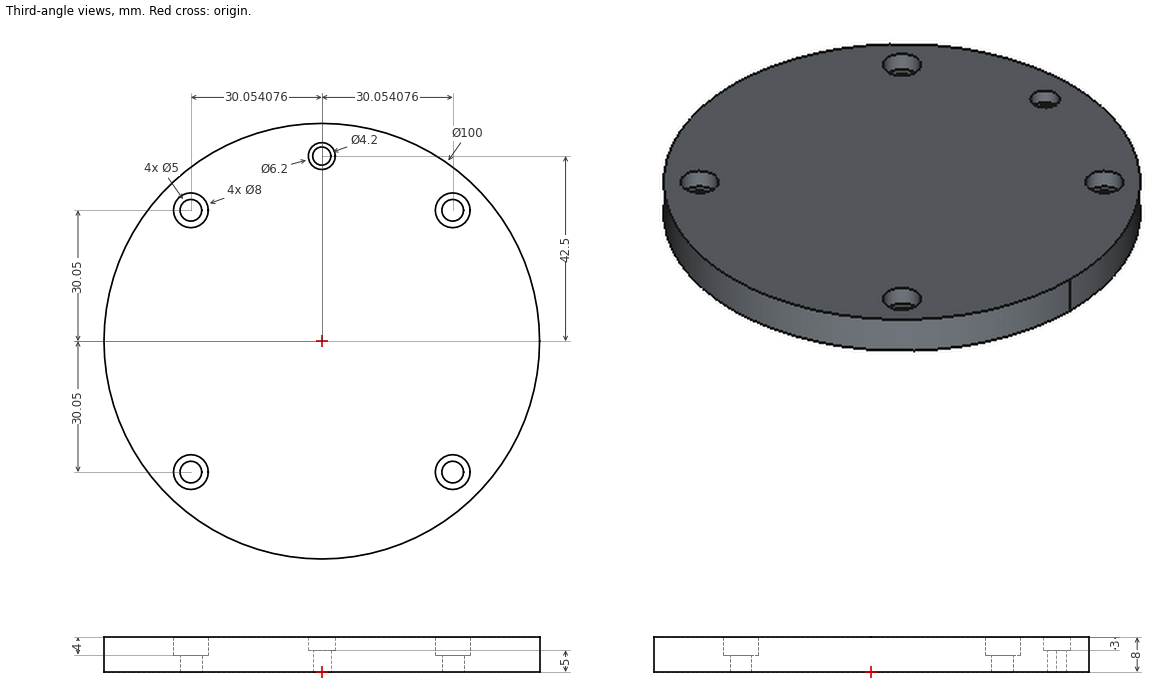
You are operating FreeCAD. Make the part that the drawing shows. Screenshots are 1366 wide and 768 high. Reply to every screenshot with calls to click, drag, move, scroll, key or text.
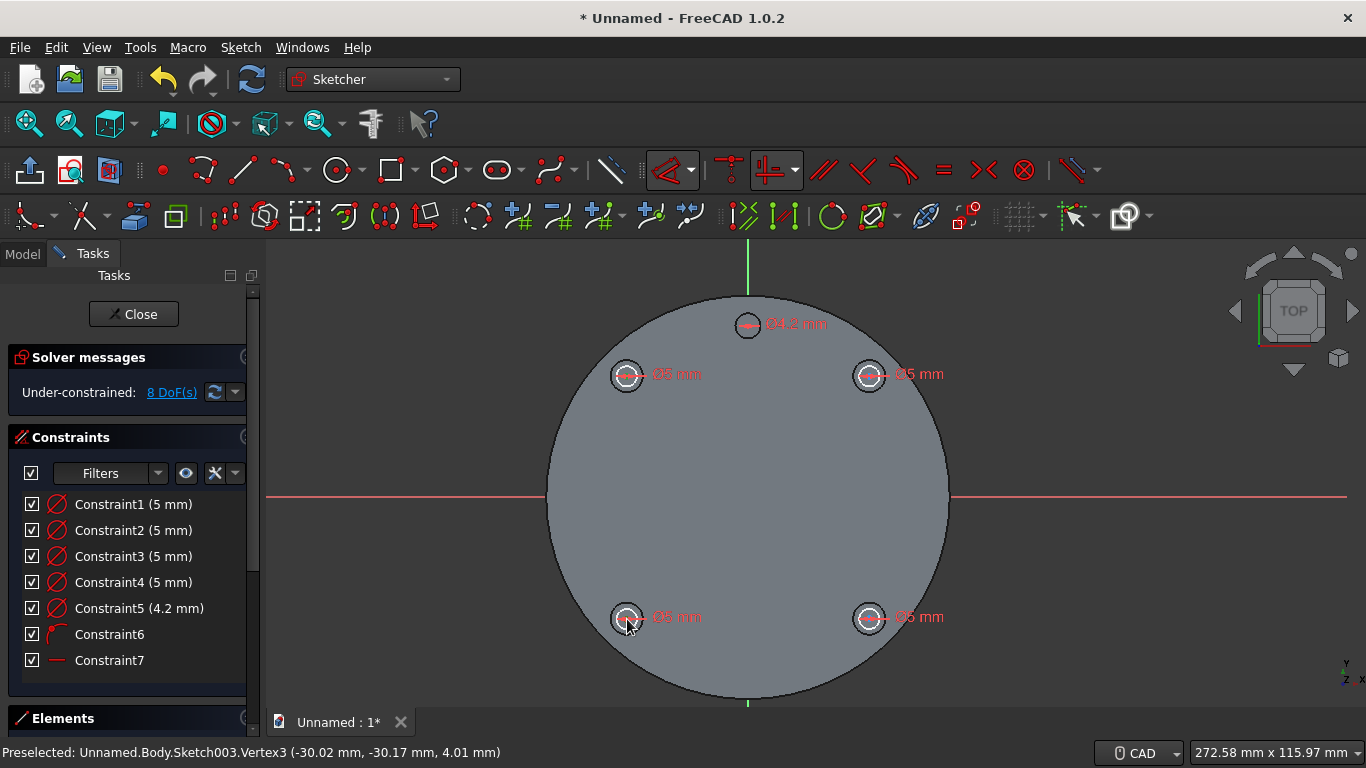
key(v)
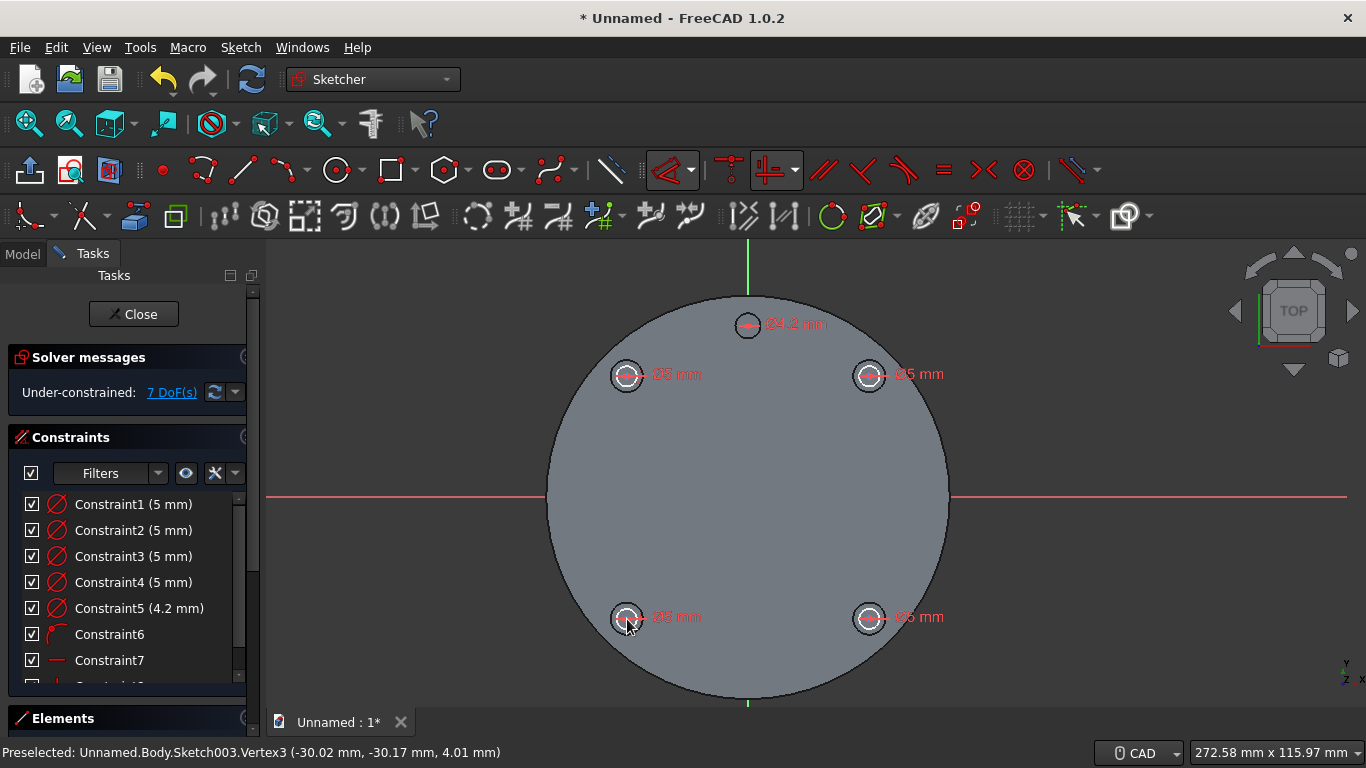
click(869, 376)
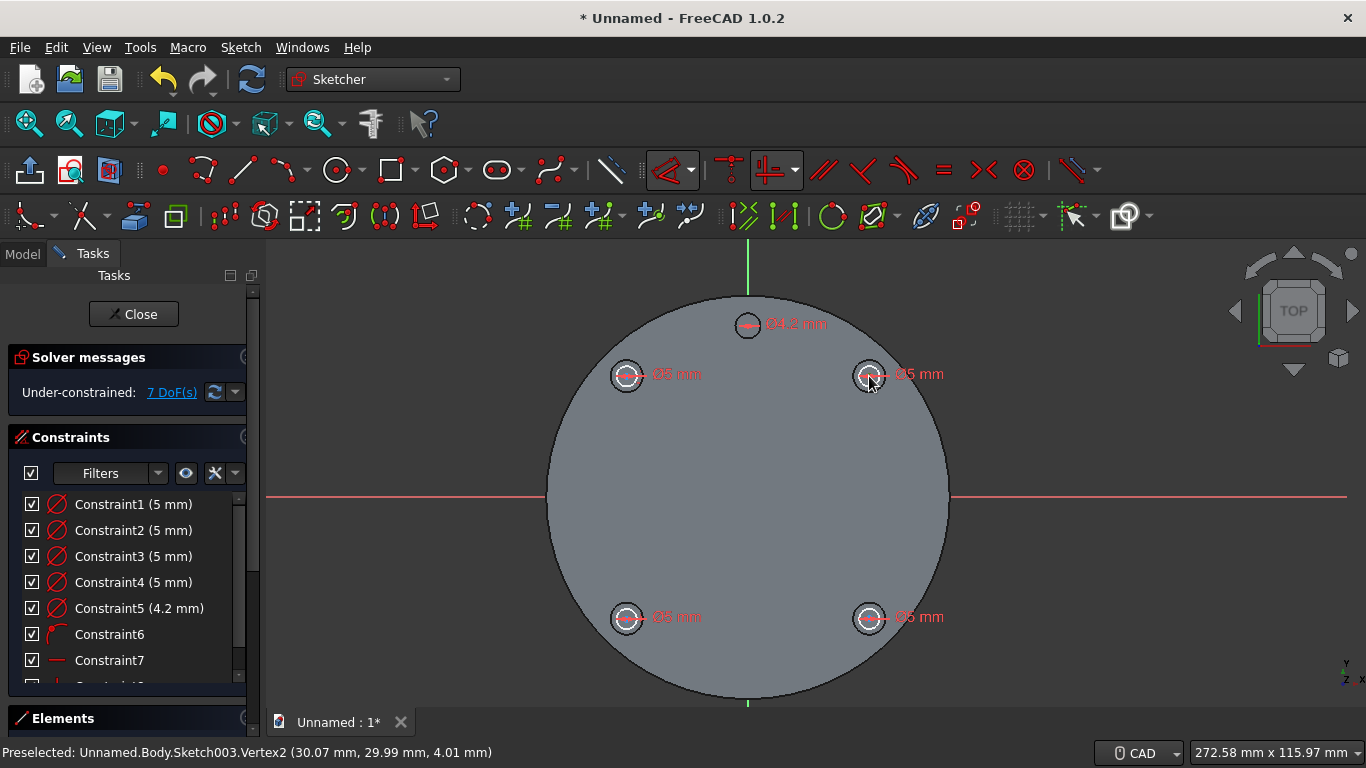
click(869, 619)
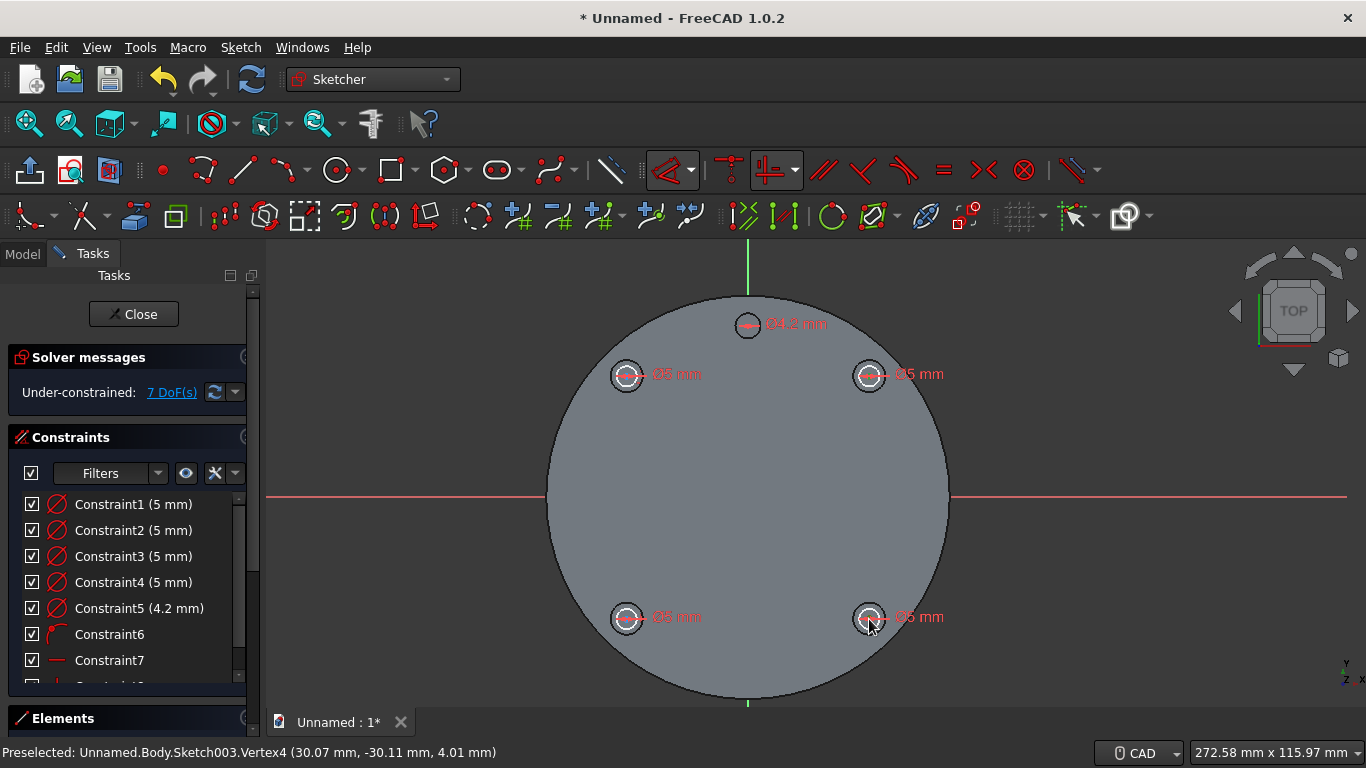
key(v)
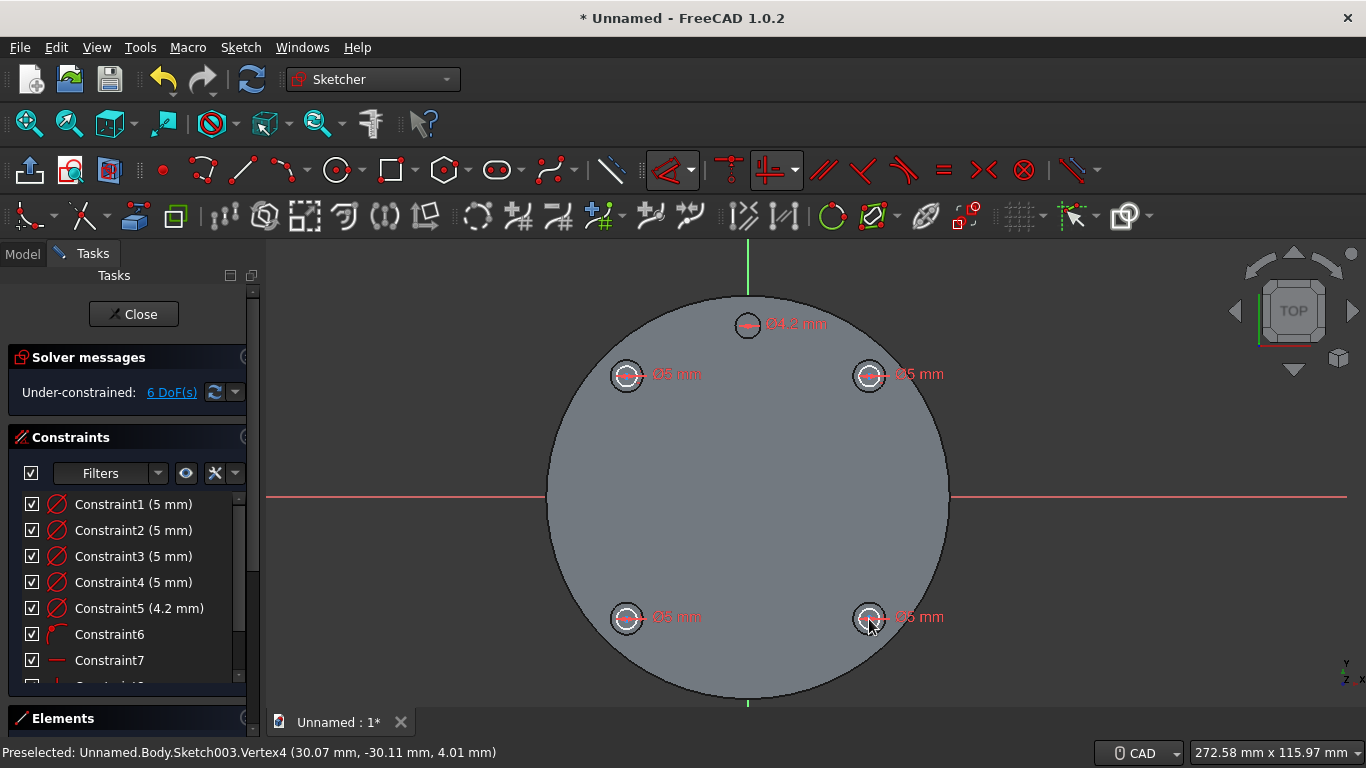
click(627, 619)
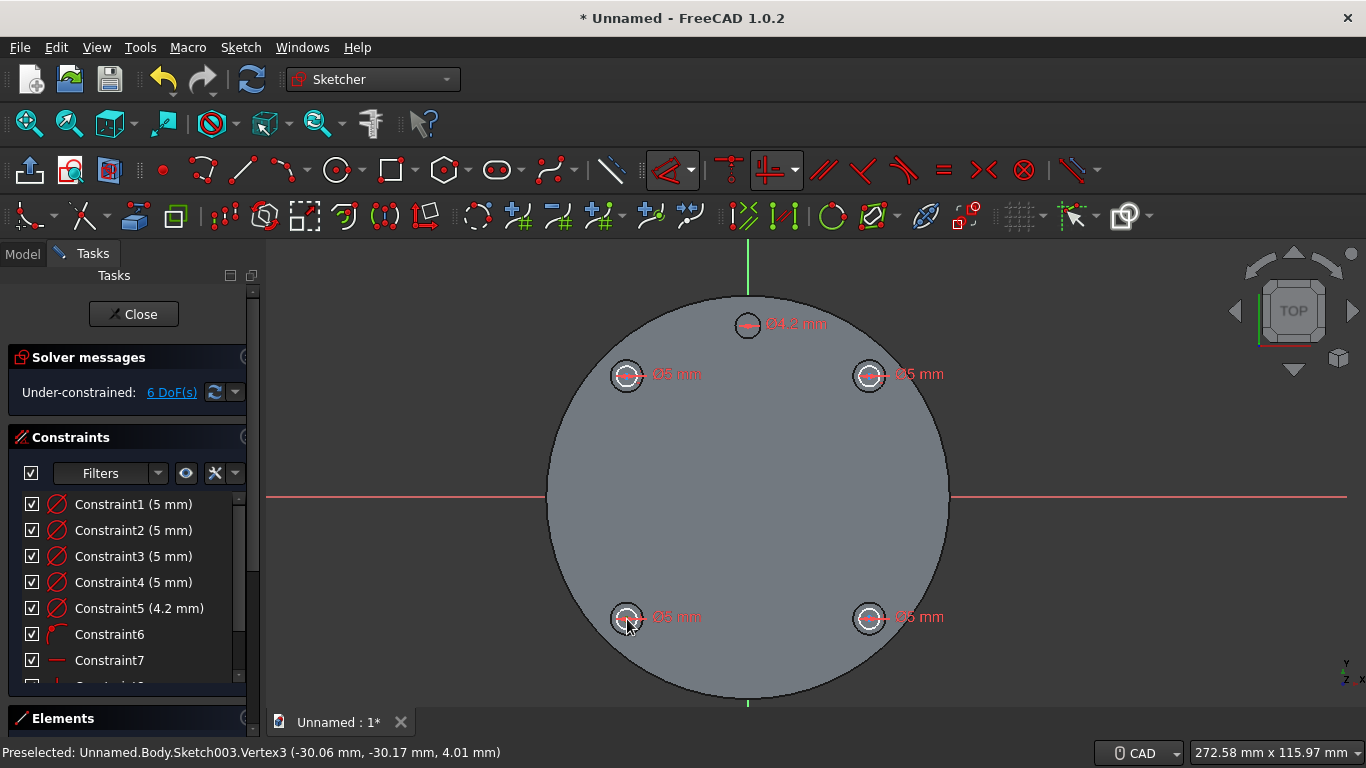
click(869, 619)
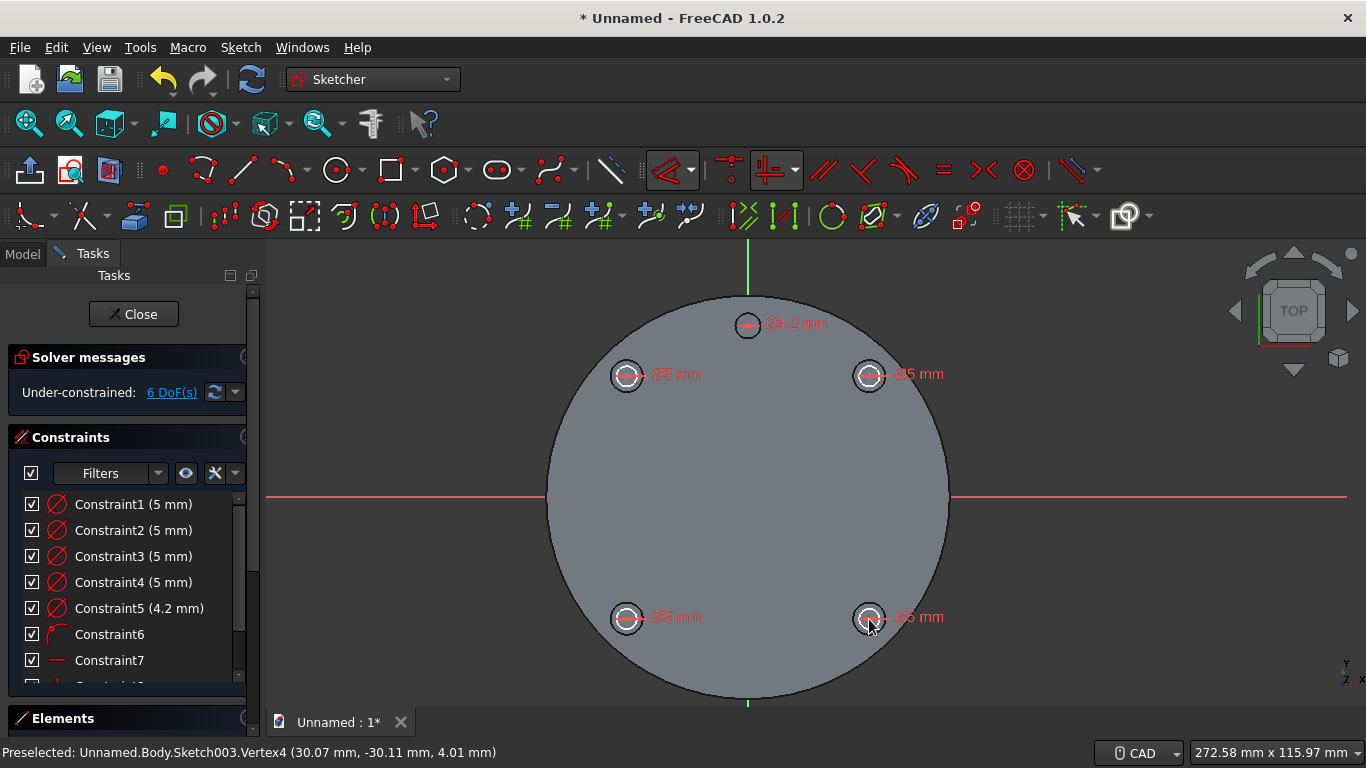
key(h)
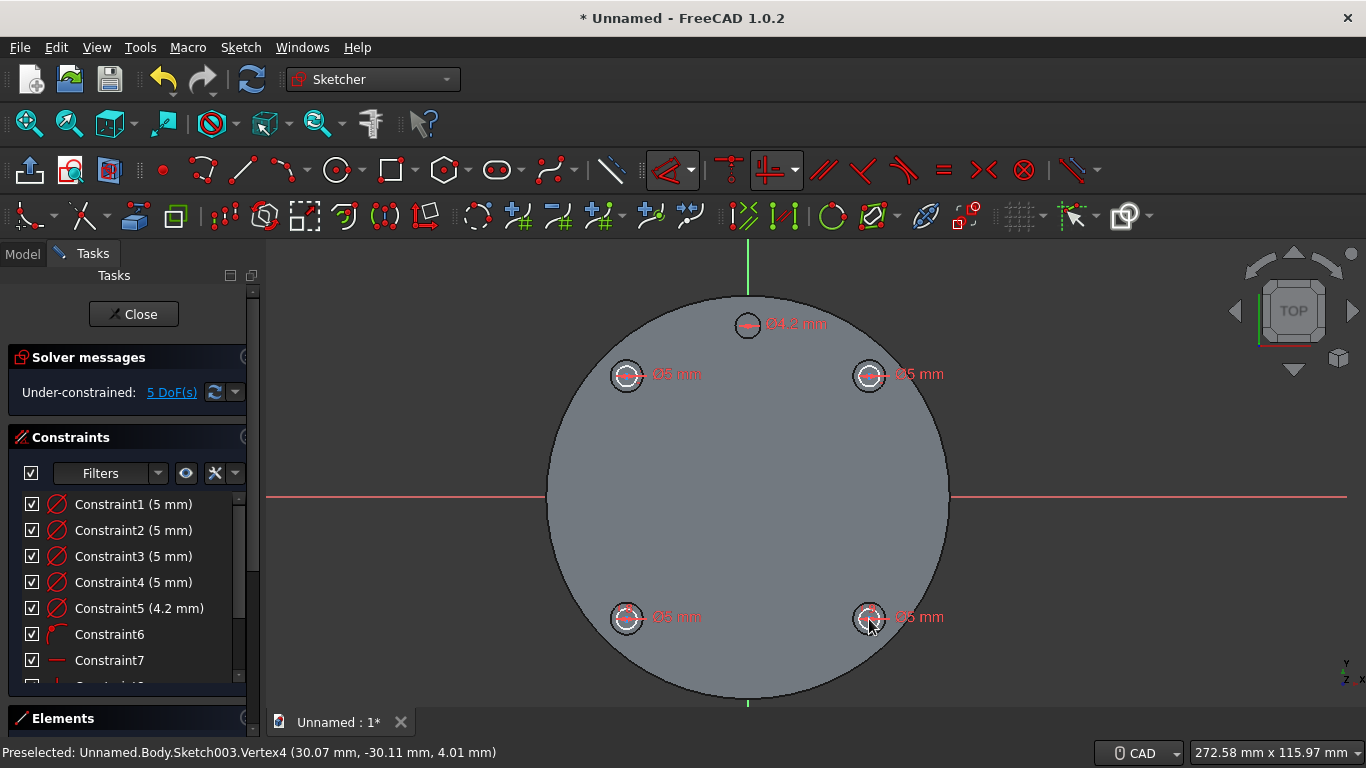
click(748, 326)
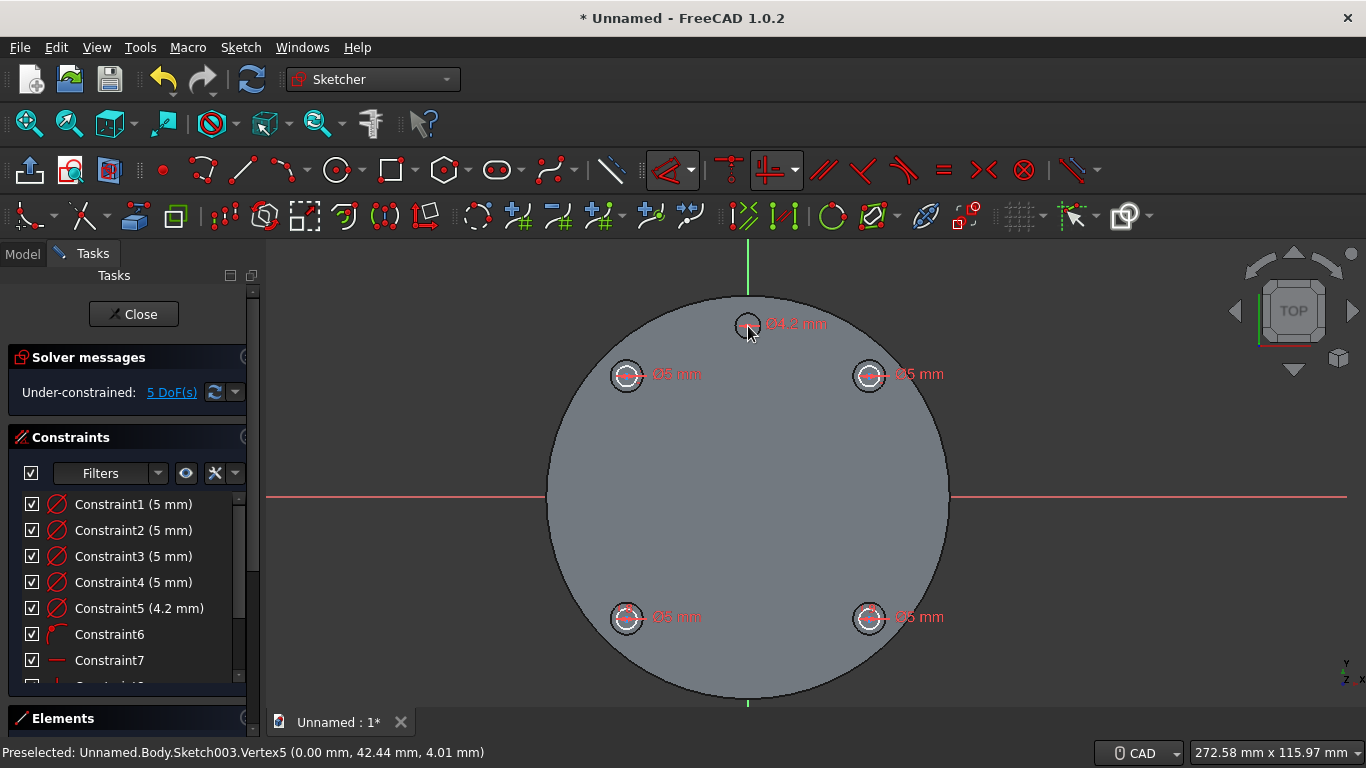
click(694, 170)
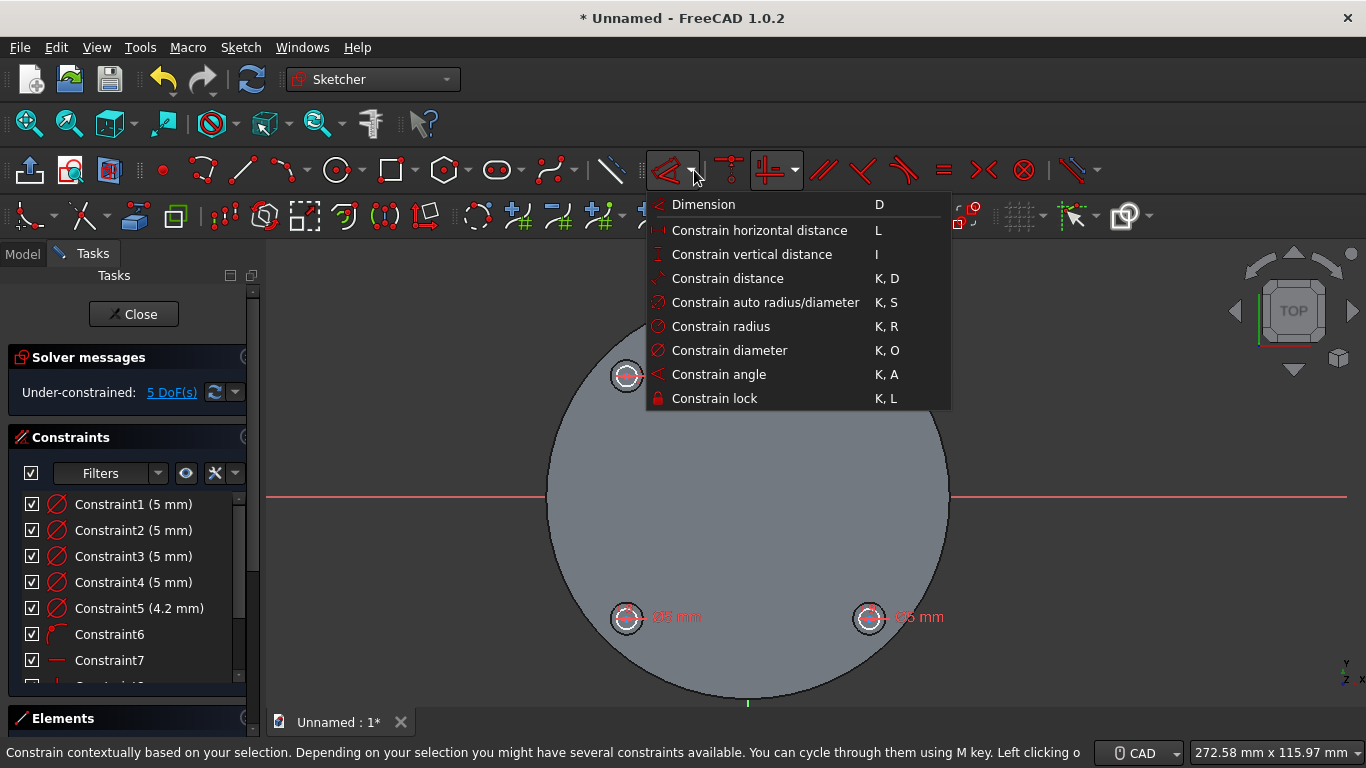
click(799, 254)